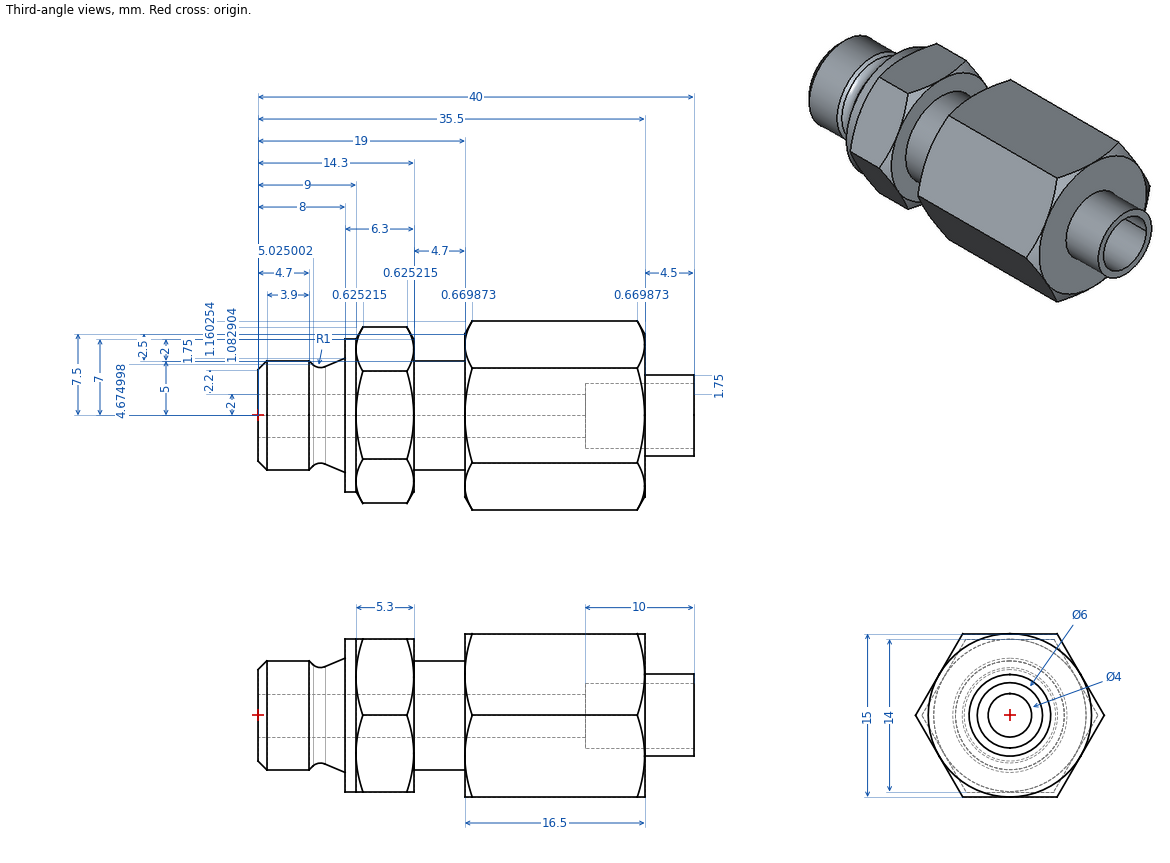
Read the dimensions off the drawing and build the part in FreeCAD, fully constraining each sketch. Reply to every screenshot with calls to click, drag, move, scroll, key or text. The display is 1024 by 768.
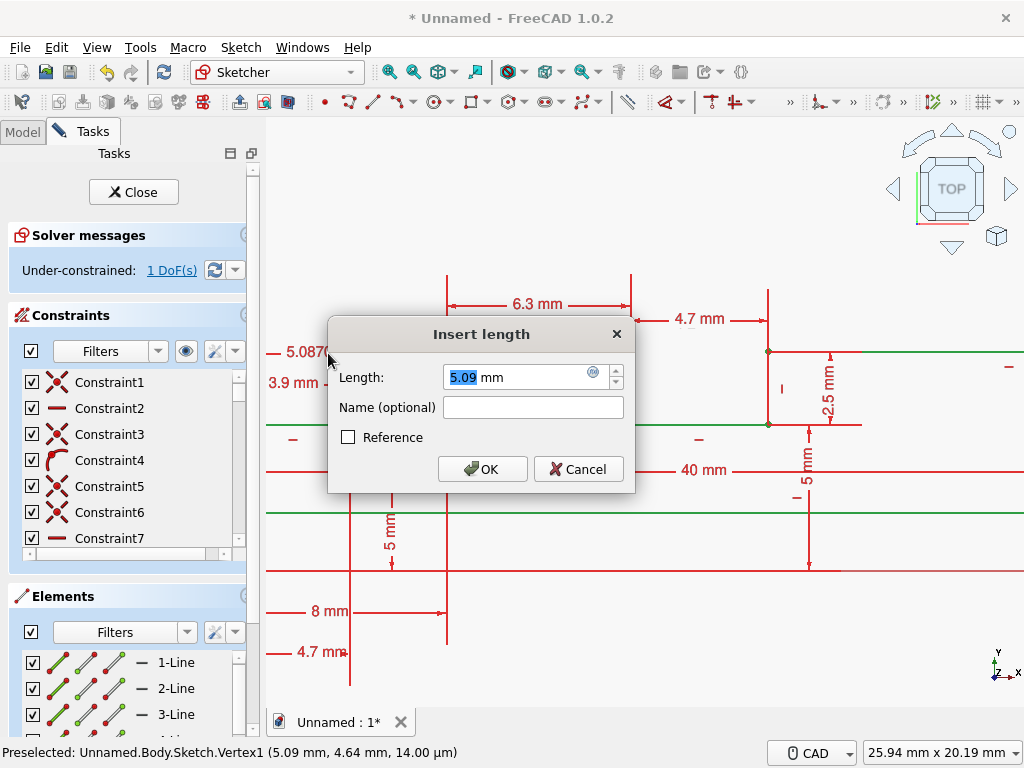
text(5.025002)
key(Return)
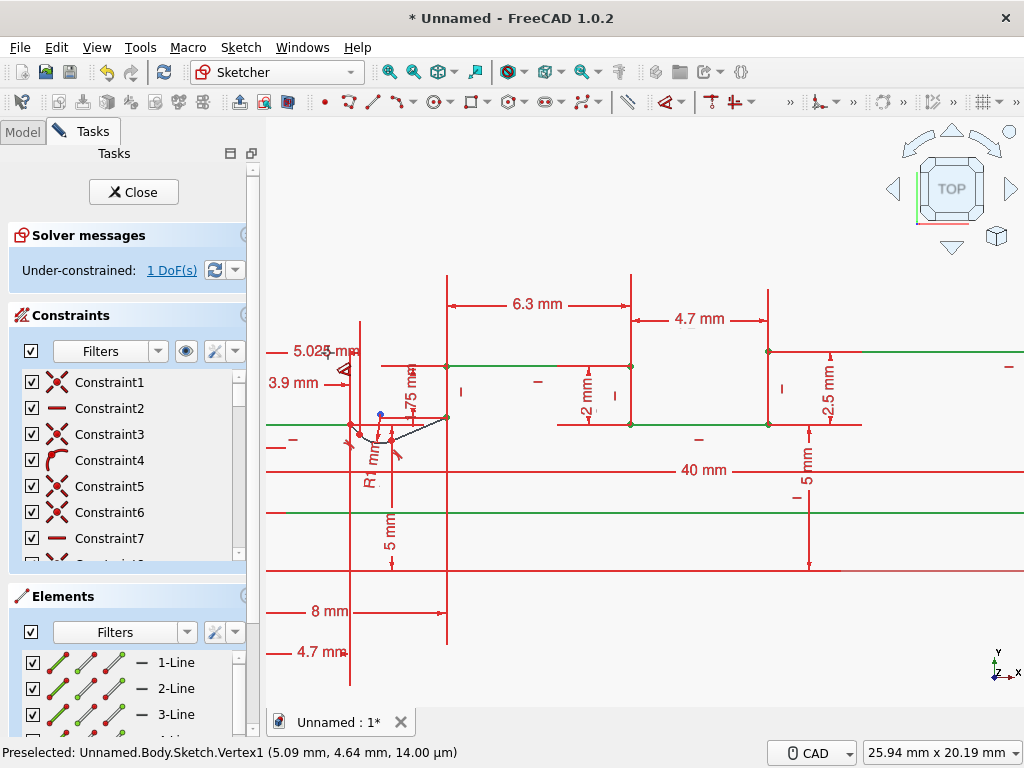
click(360, 435)
click(466, 471)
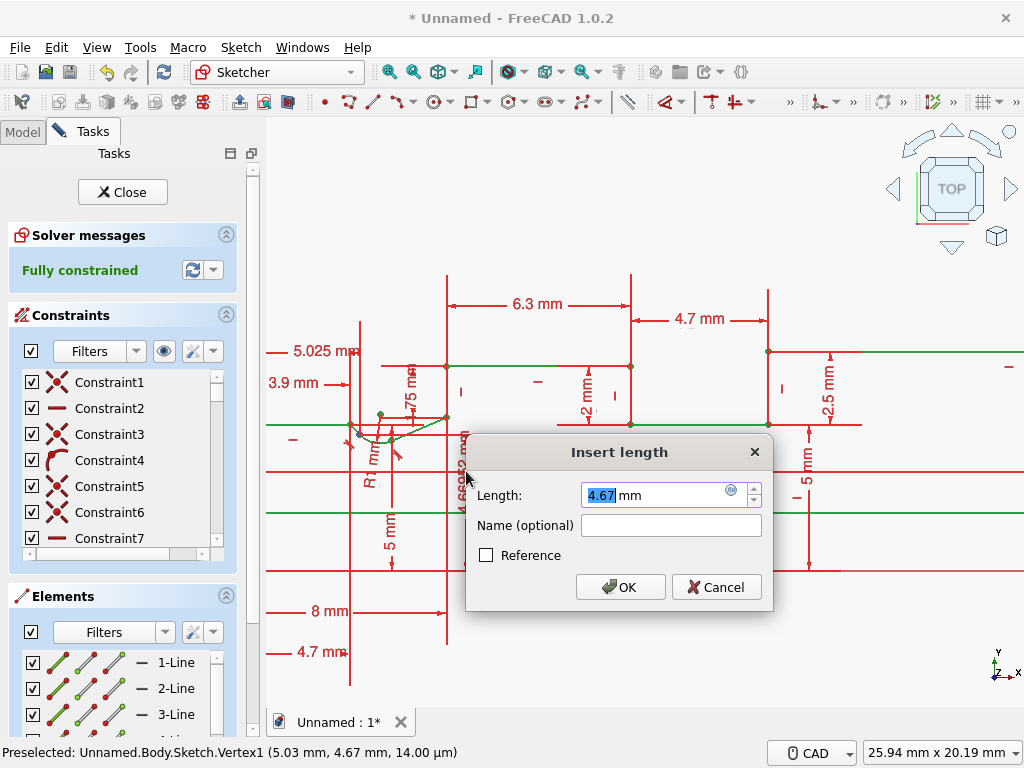
text(4.674998)
key(Return)
key(Escape)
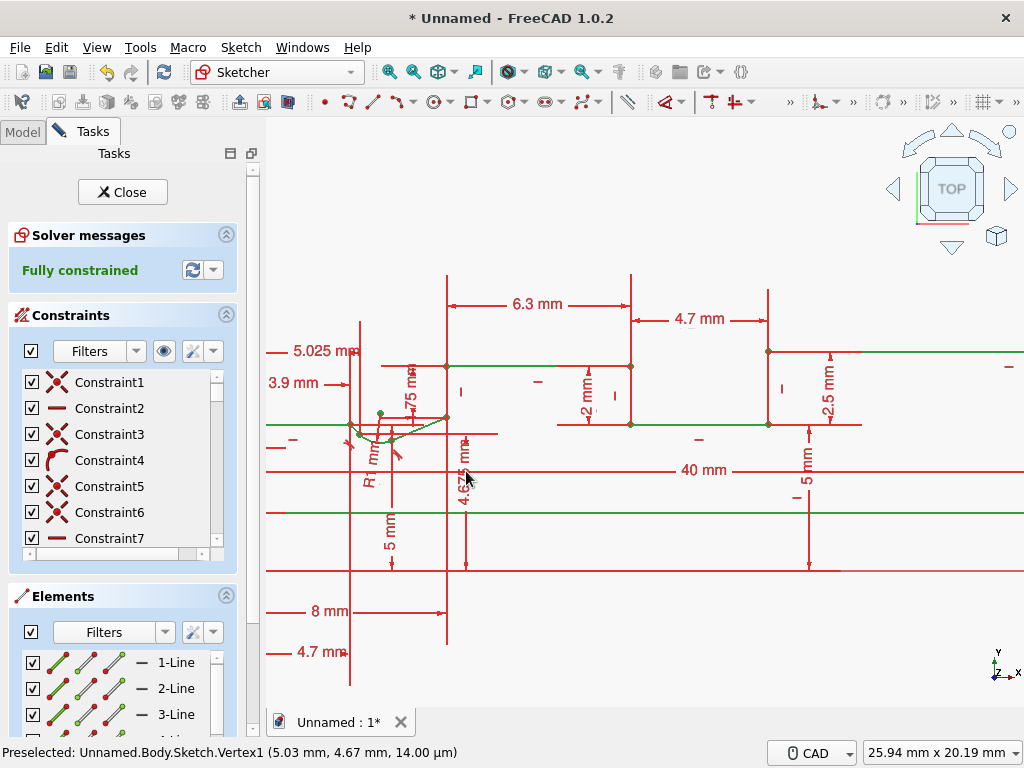
click(123, 192)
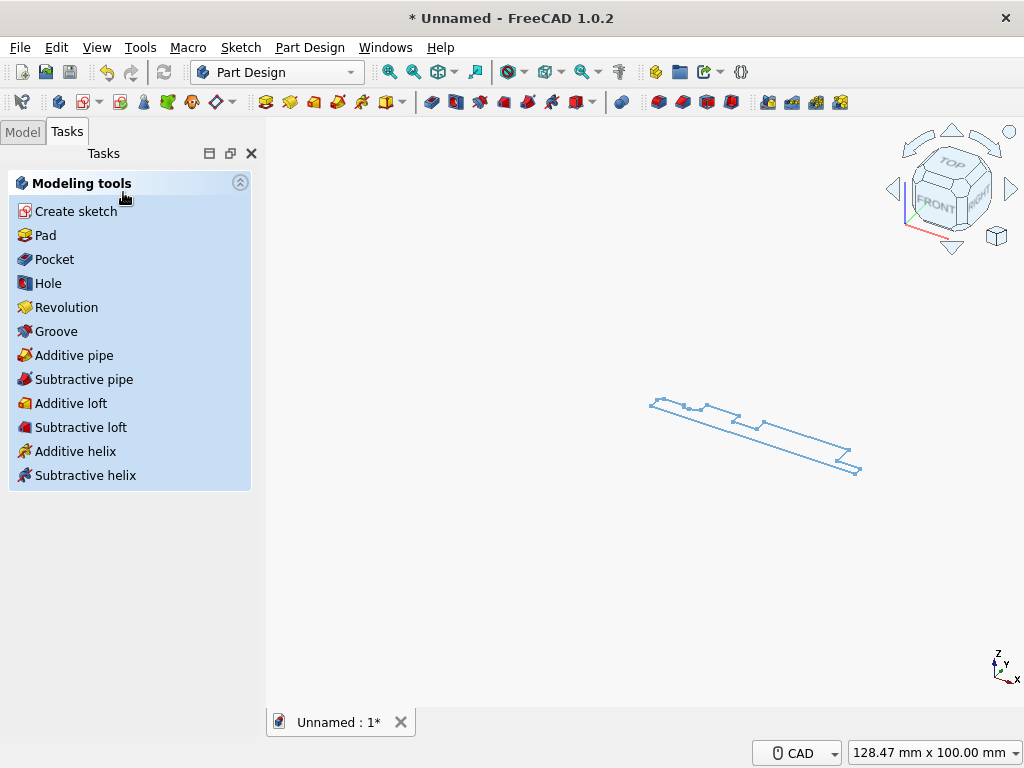
click(290, 102)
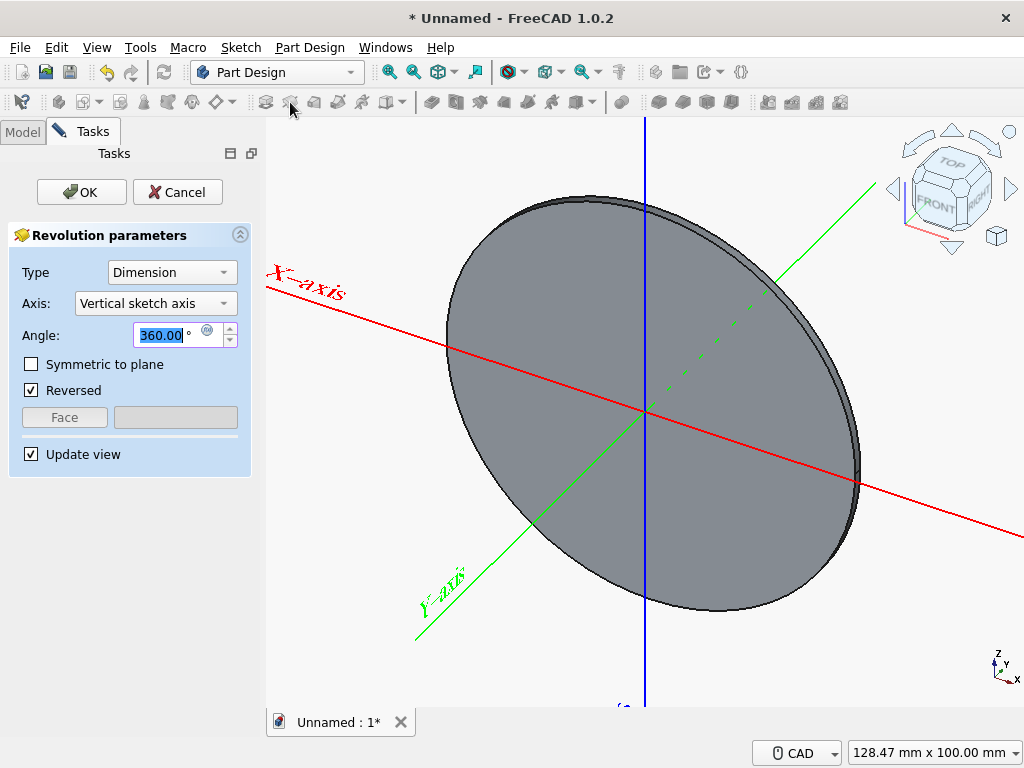
click(156, 304)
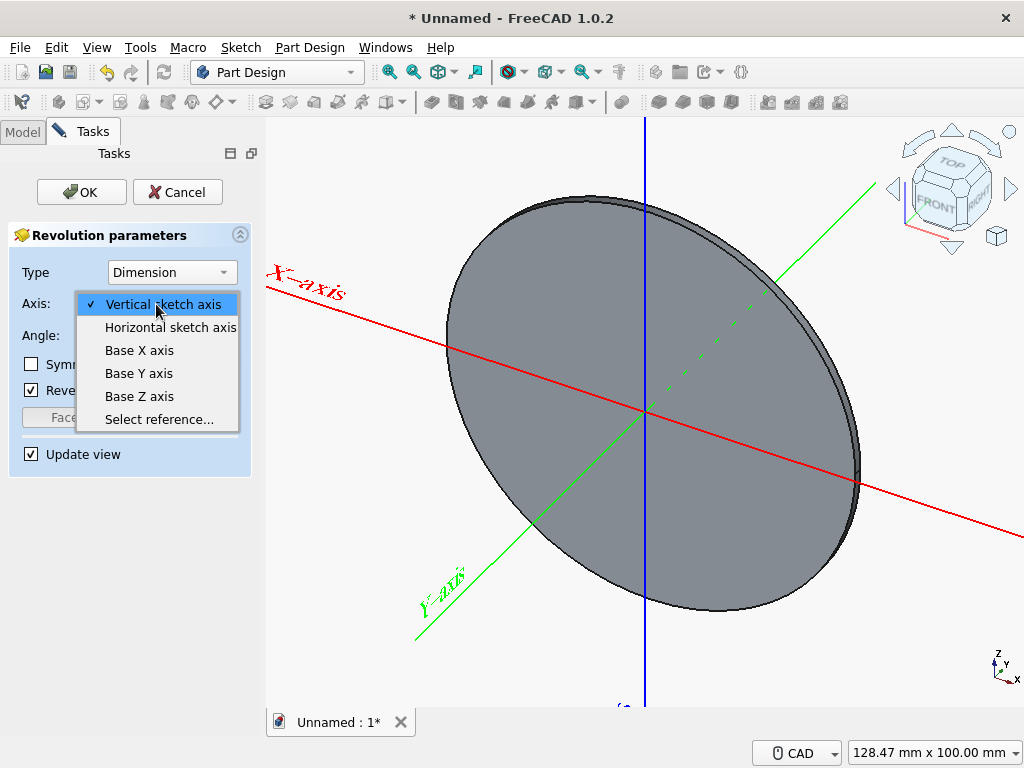
click(156, 328)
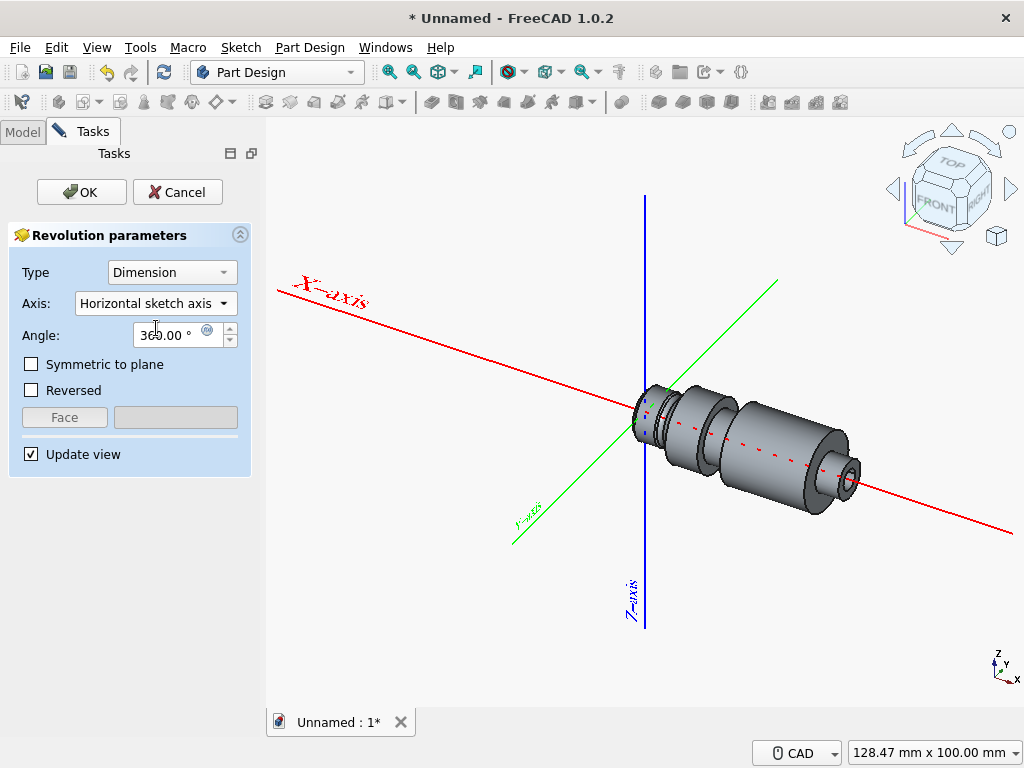
click(82, 192)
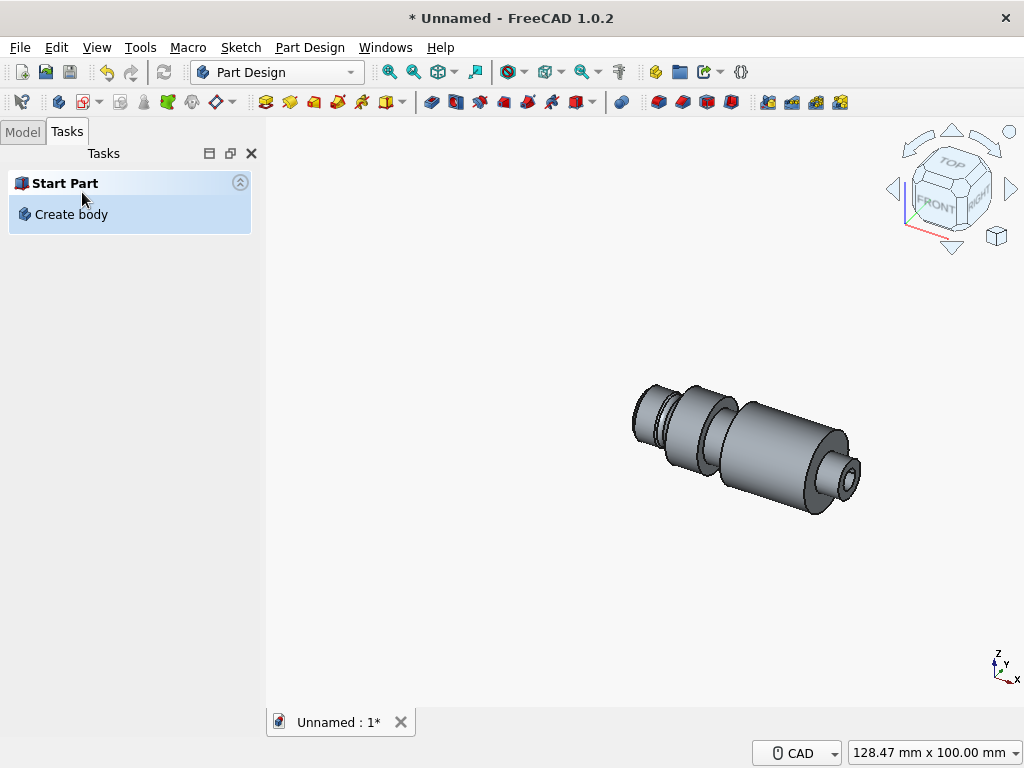
key(v)
key(f)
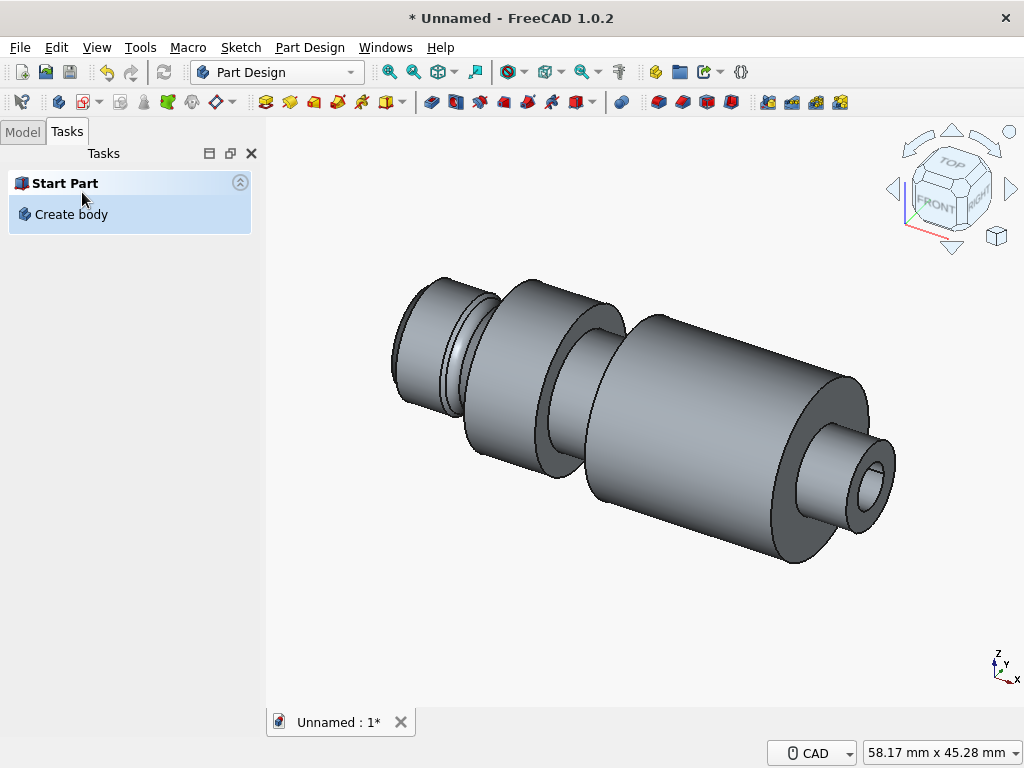
click(23, 131)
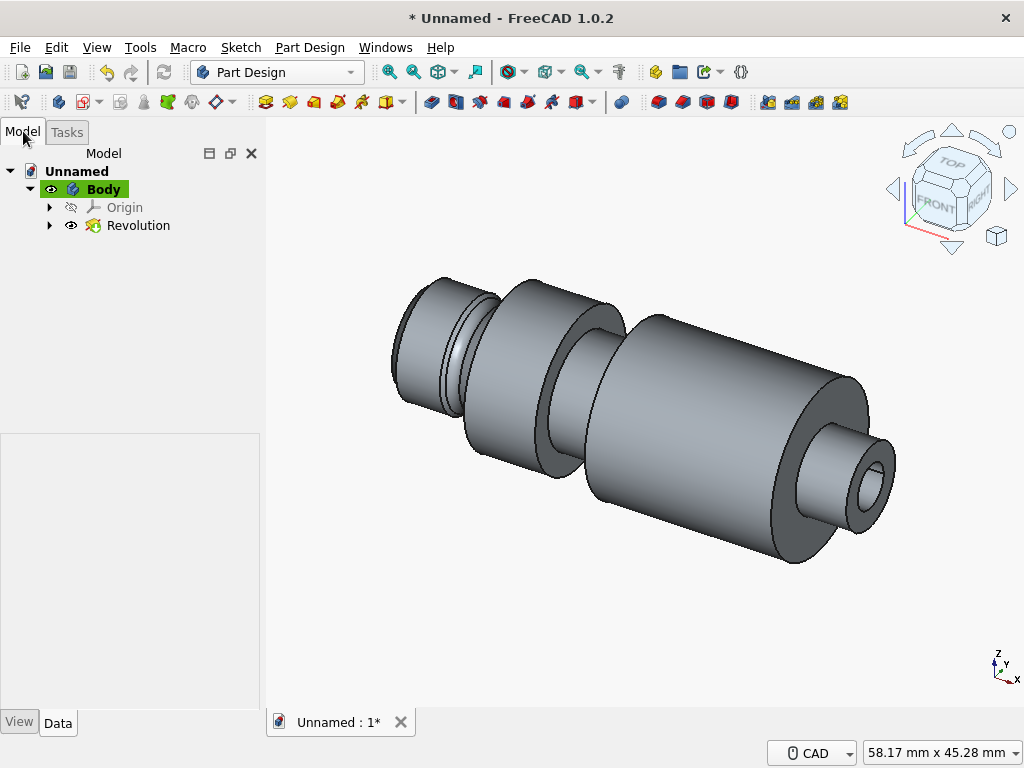
click(50, 207)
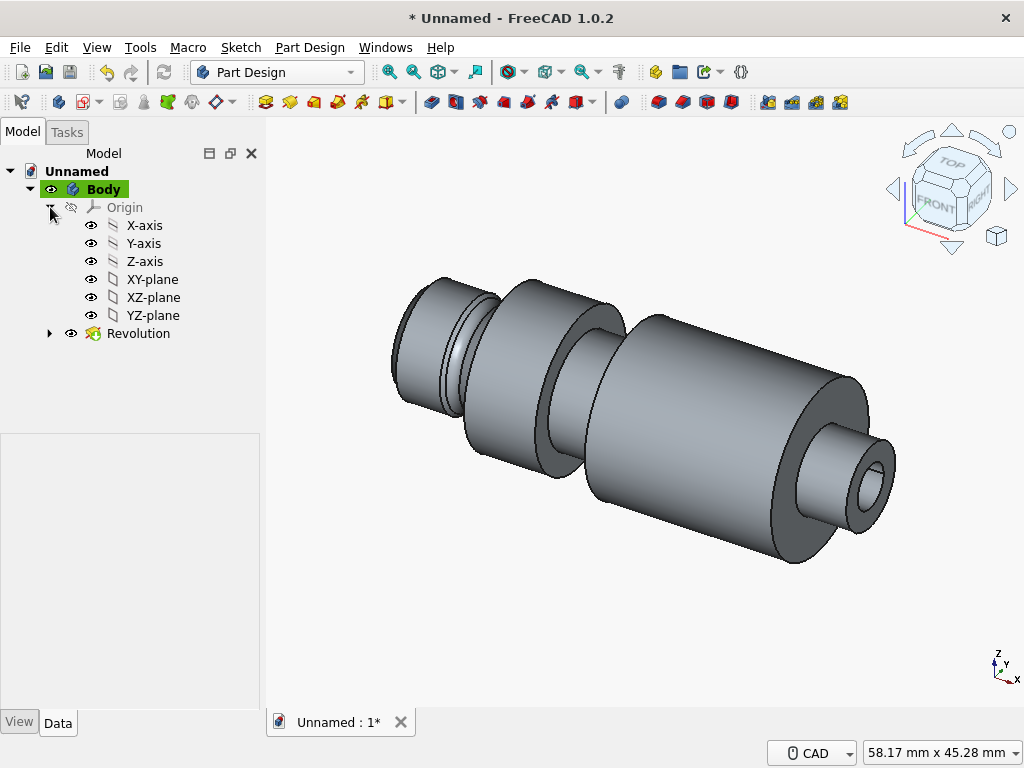
click(136, 315)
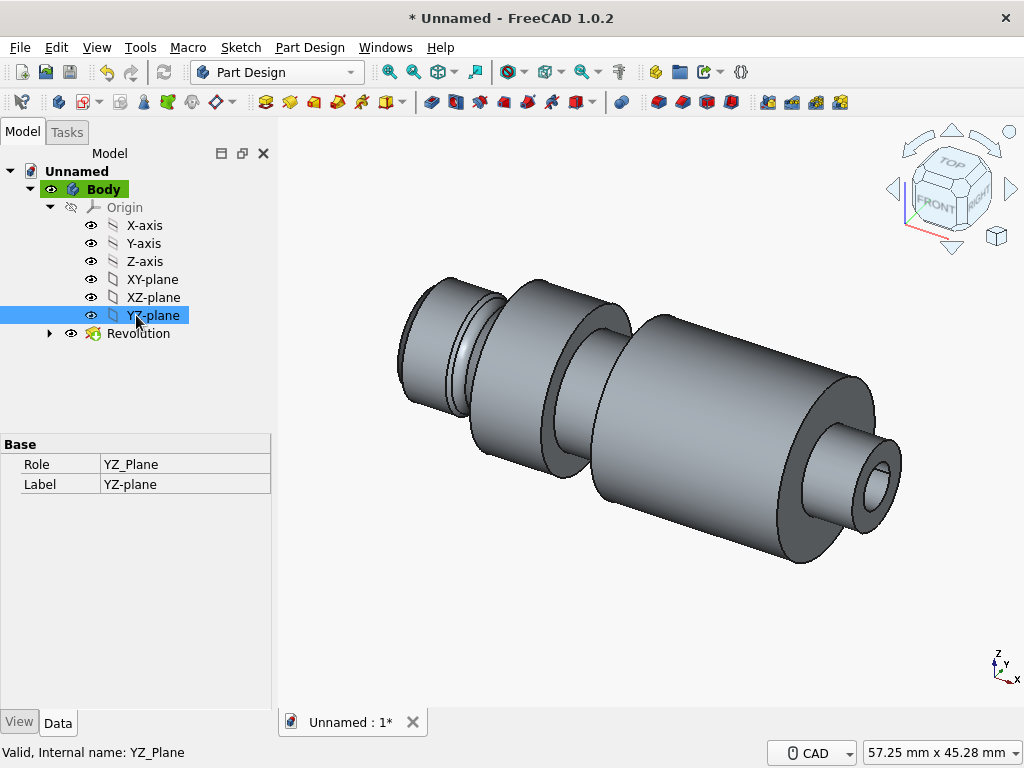
click(216, 102)